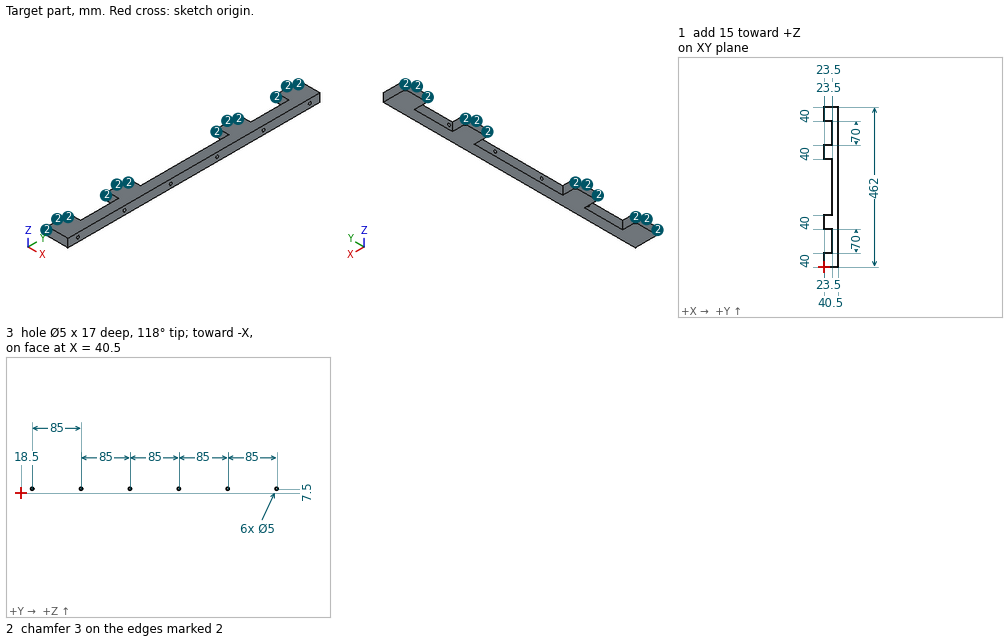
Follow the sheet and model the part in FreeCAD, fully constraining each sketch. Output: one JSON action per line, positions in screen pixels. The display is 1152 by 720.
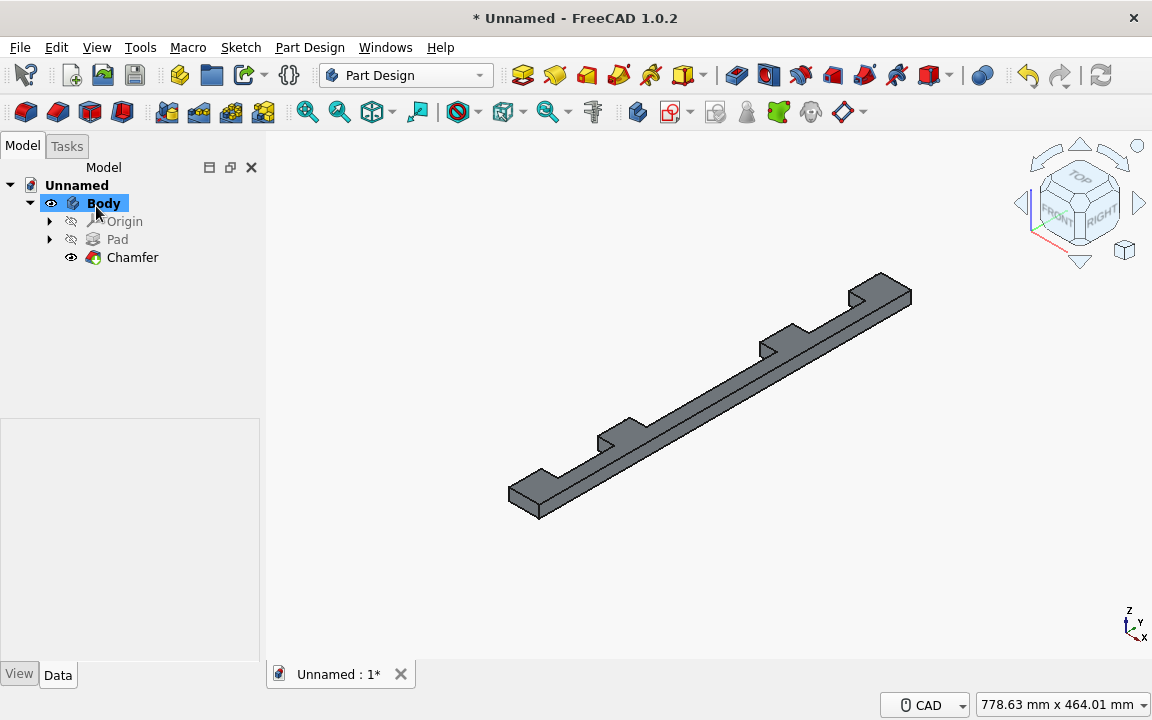
{"action": "key", "text": "3"}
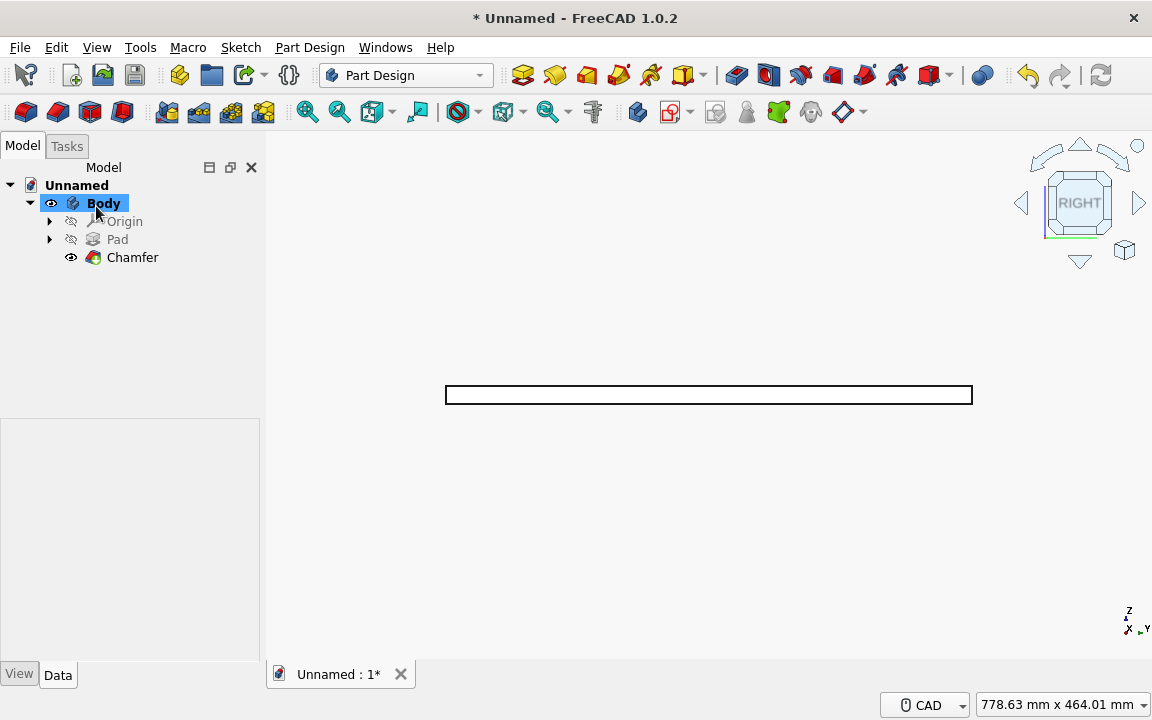
{"action": "left_click", "coordinate": [934, 394]}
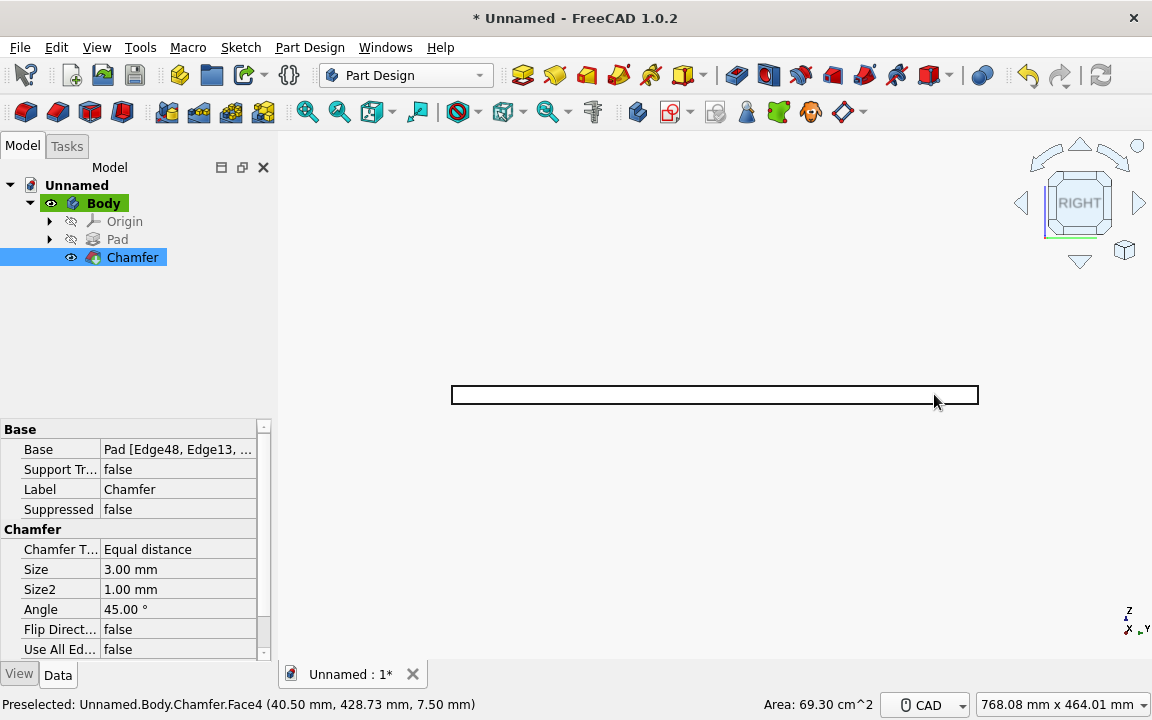
{"action": "left_click", "coordinate": [670, 112]}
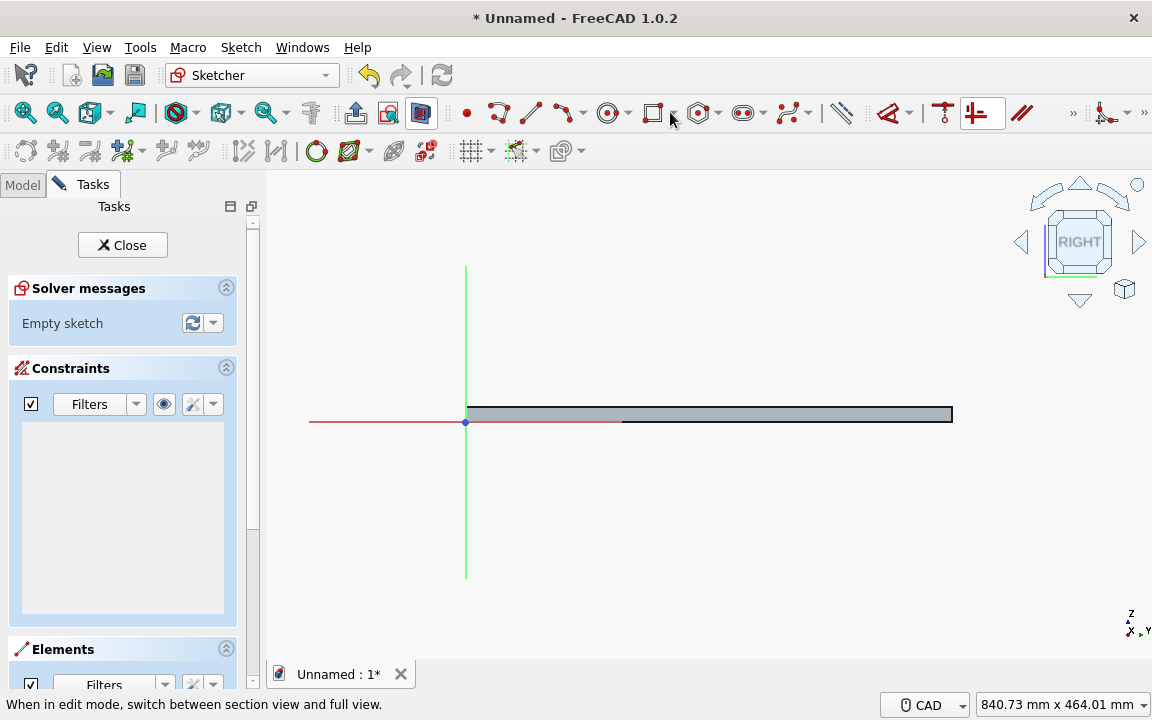
{"action": "left_click", "coordinate": [608, 114]}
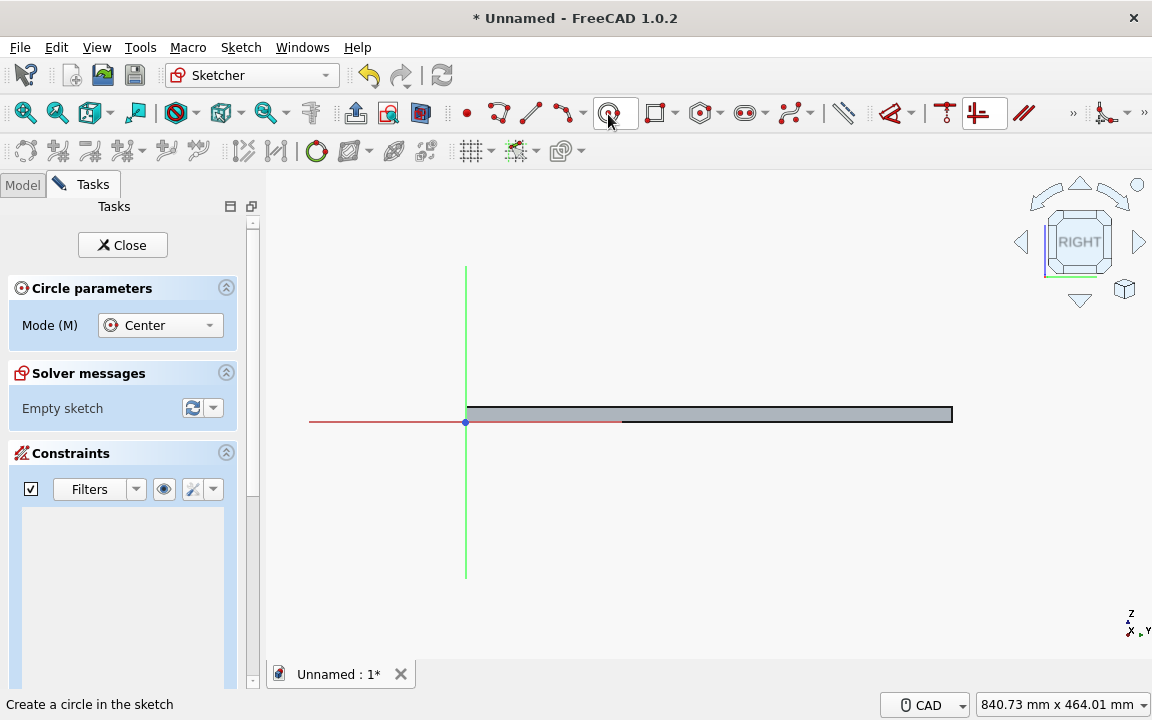
{"action": "scroll", "coordinate": [933, 414], "scroll_direction": "up", "scroll_amount": 11}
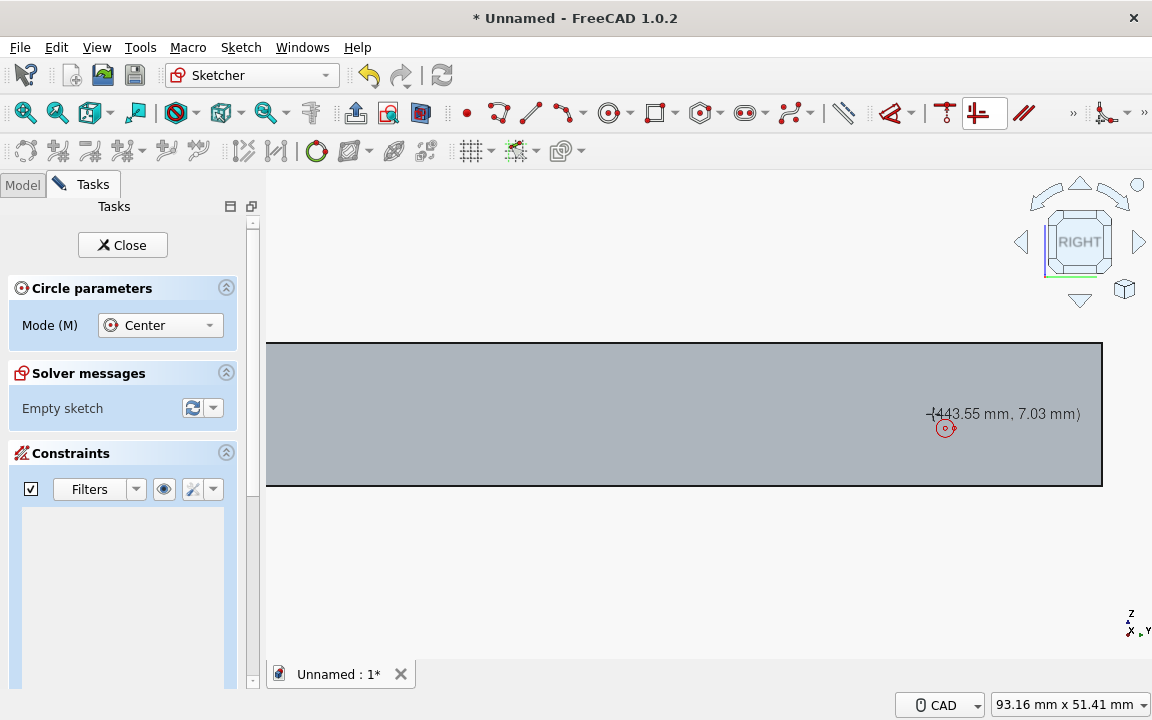
{"action": "scroll", "coordinate": [866, 412], "scroll_direction": "down", "scroll_amount": 11}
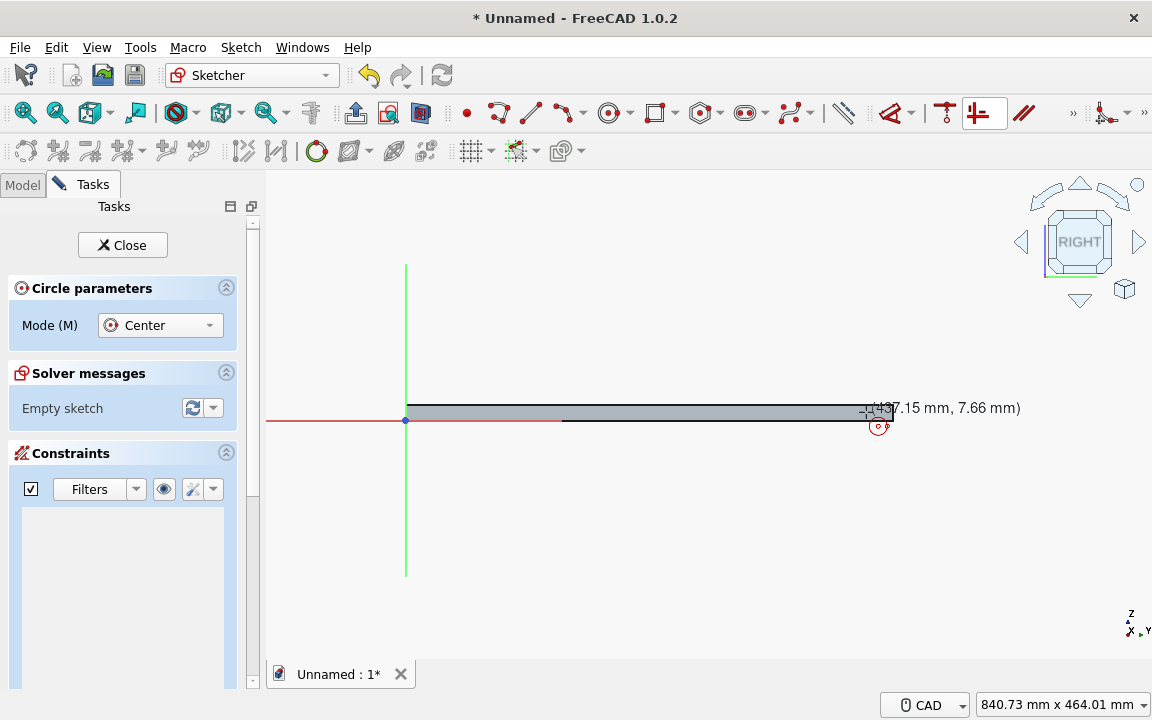
{"action": "scroll", "coordinate": [873, 413], "scroll_direction": "up", "scroll_amount": 4}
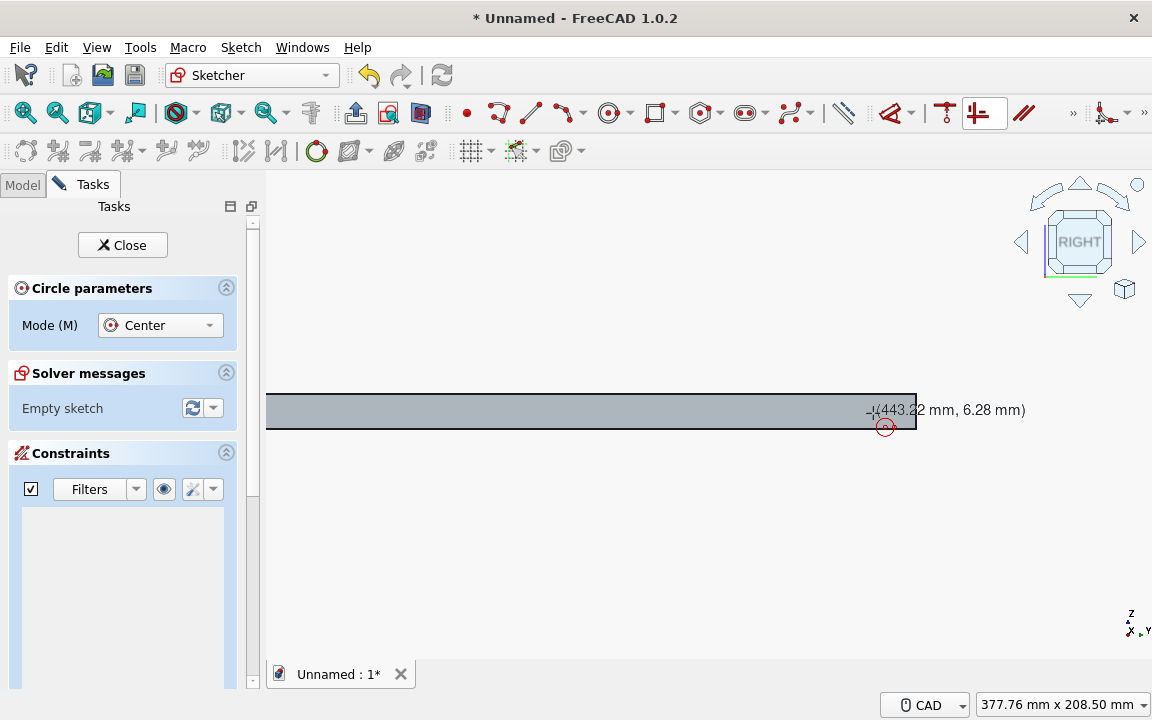
{"action": "left_click", "coordinate": [873, 412]}
{"action": "mouse_move", "coordinate": [877, 408]}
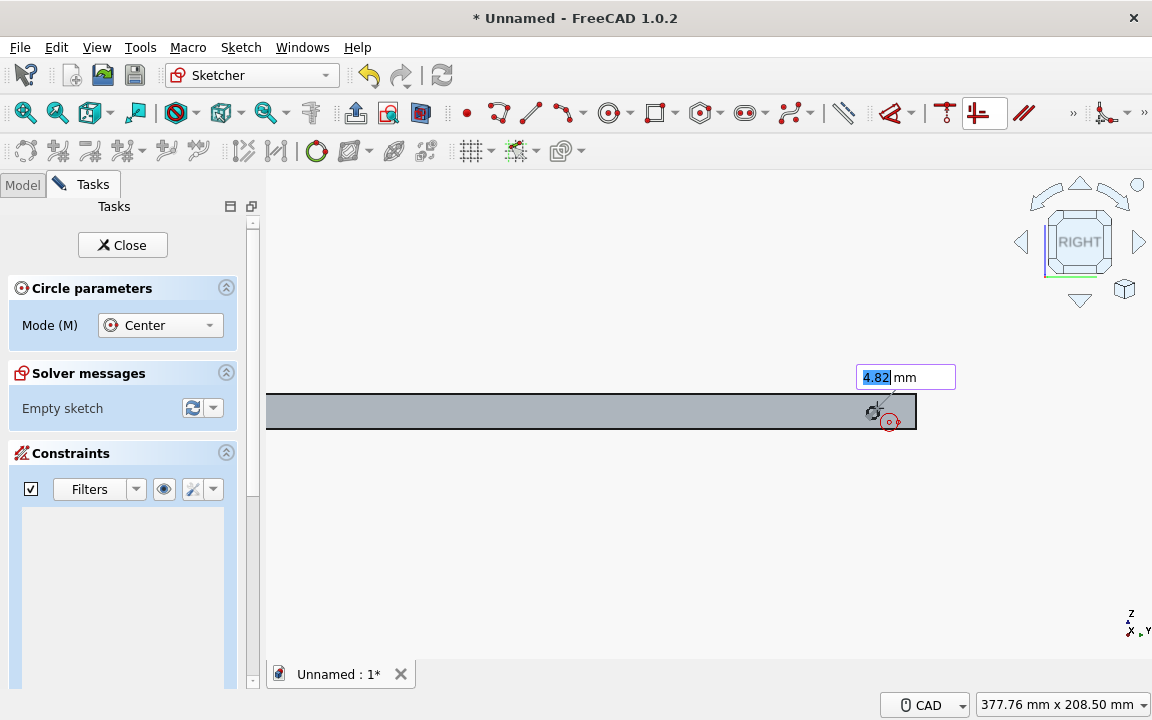
{"action": "type", "text": "5"}
{"action": "key", "text": "Return"}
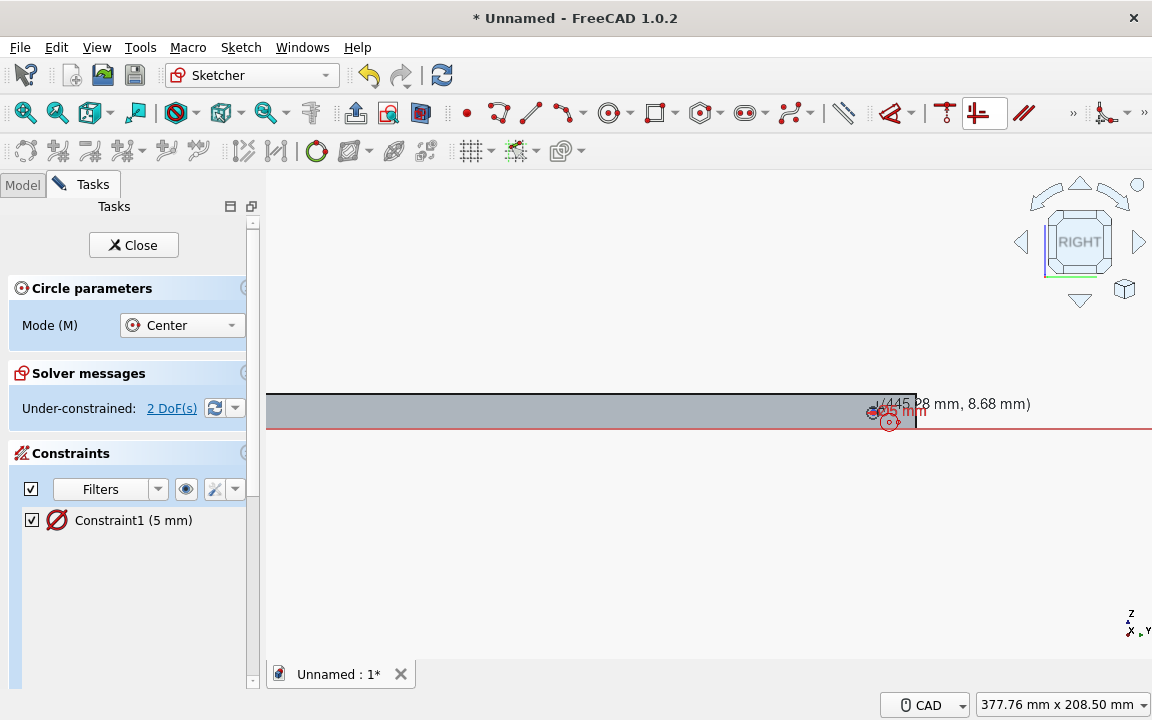
{"action": "scroll", "coordinate": [673, 412], "scroll_direction": "up", "scroll_amount": 7}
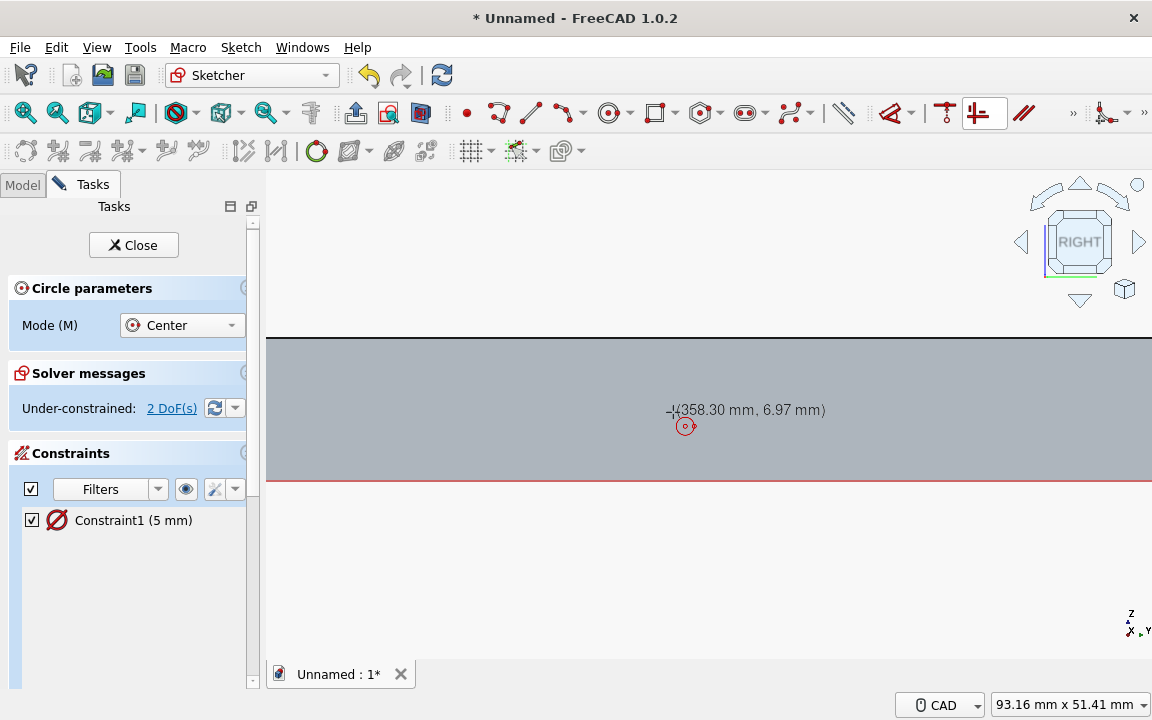
{"action": "scroll", "coordinate": [797, 412], "scroll_direction": "down", "scroll_amount": 11}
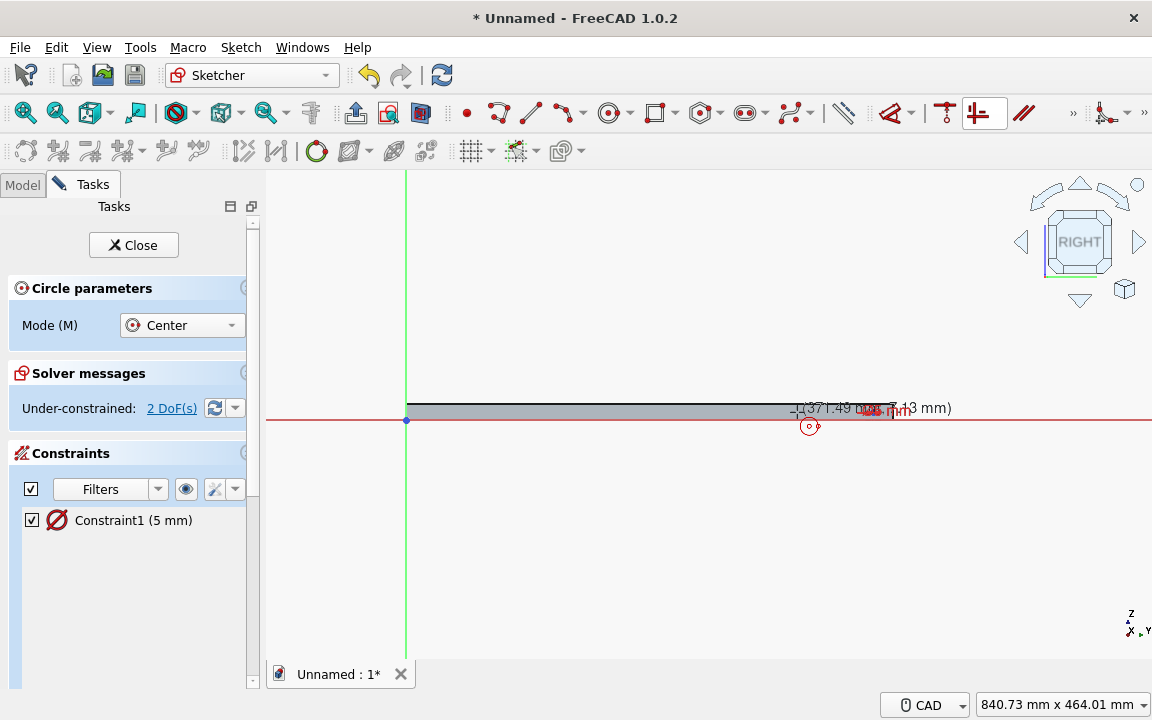
{"action": "scroll", "coordinate": [784, 412], "scroll_direction": "up", "scroll_amount": 4}